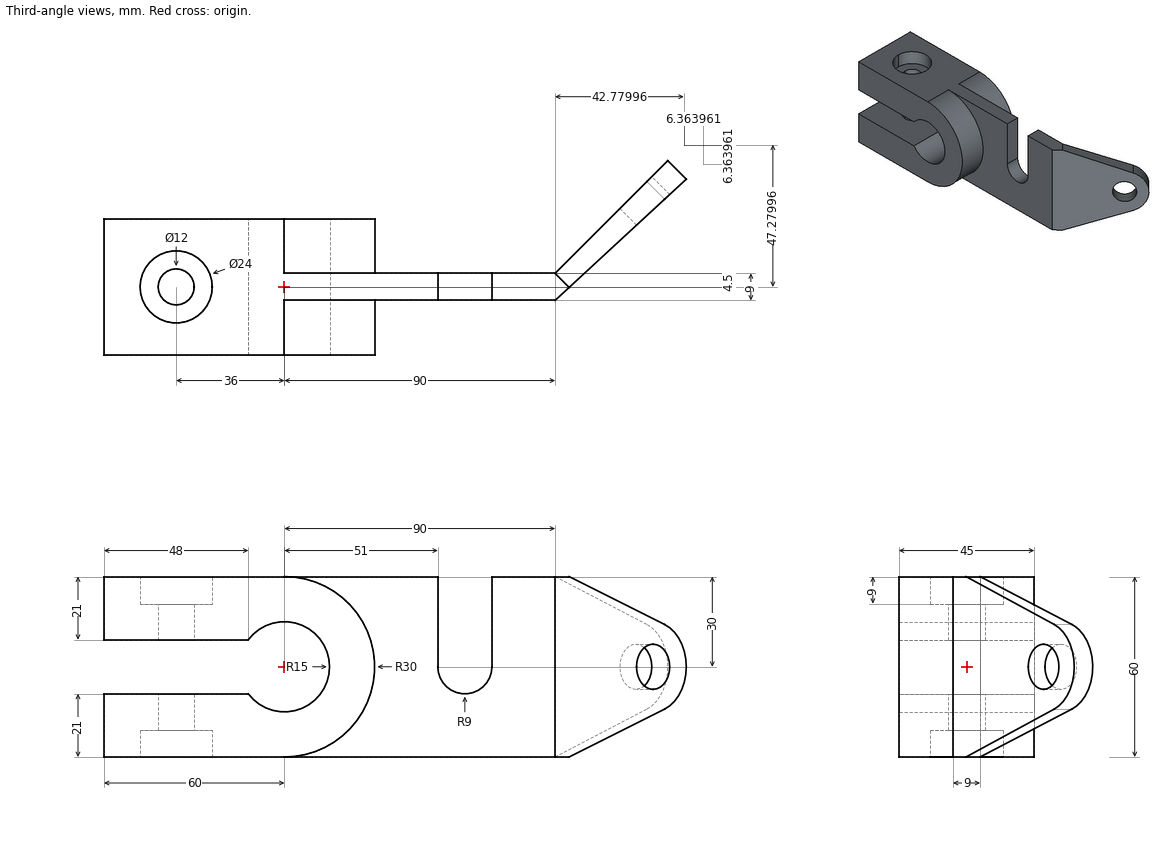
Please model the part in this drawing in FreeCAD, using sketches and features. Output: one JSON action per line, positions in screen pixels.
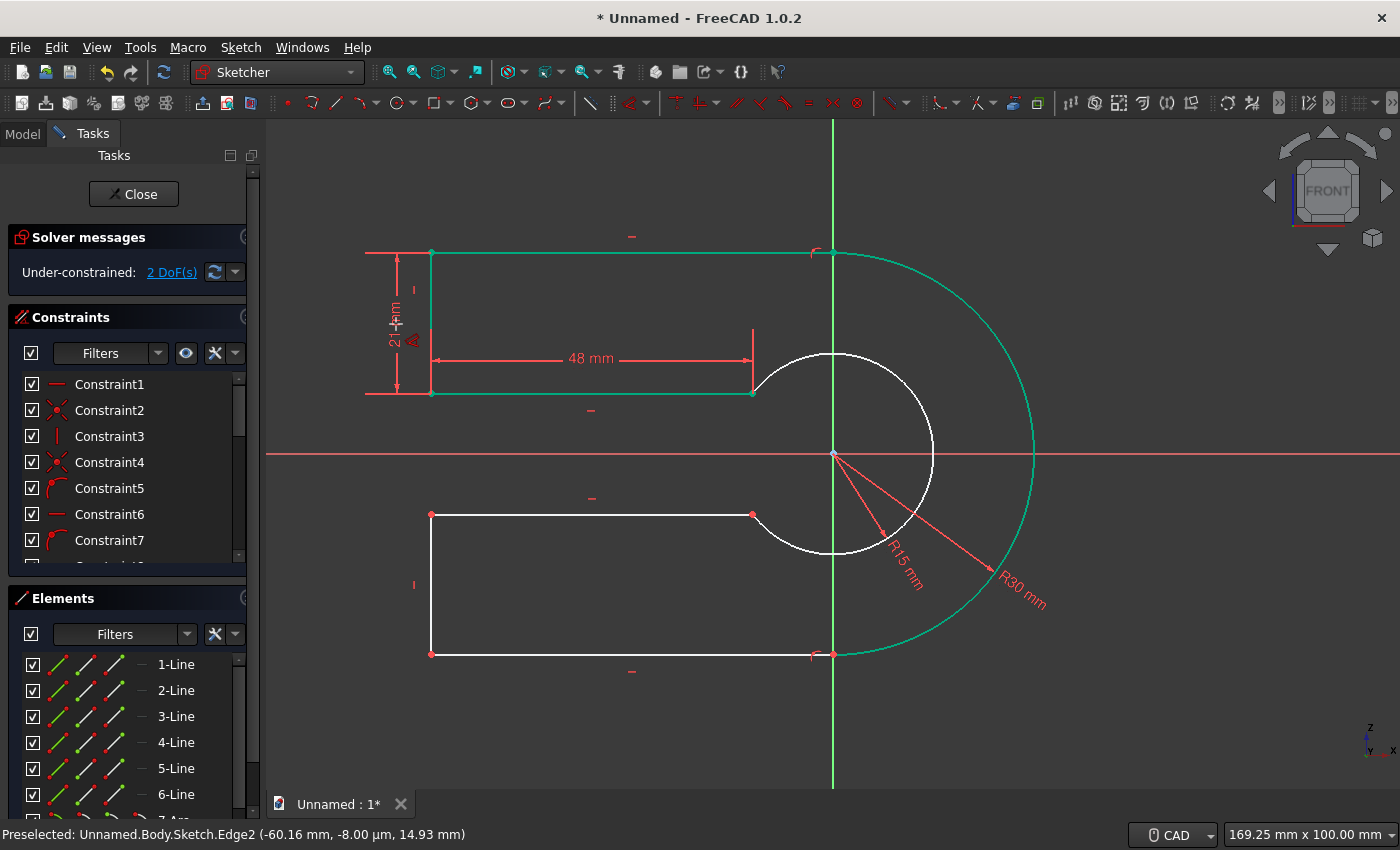
{"action": "left_click", "coordinate": [712, 655]}
{"action": "left_click", "coordinate": [632, 689]}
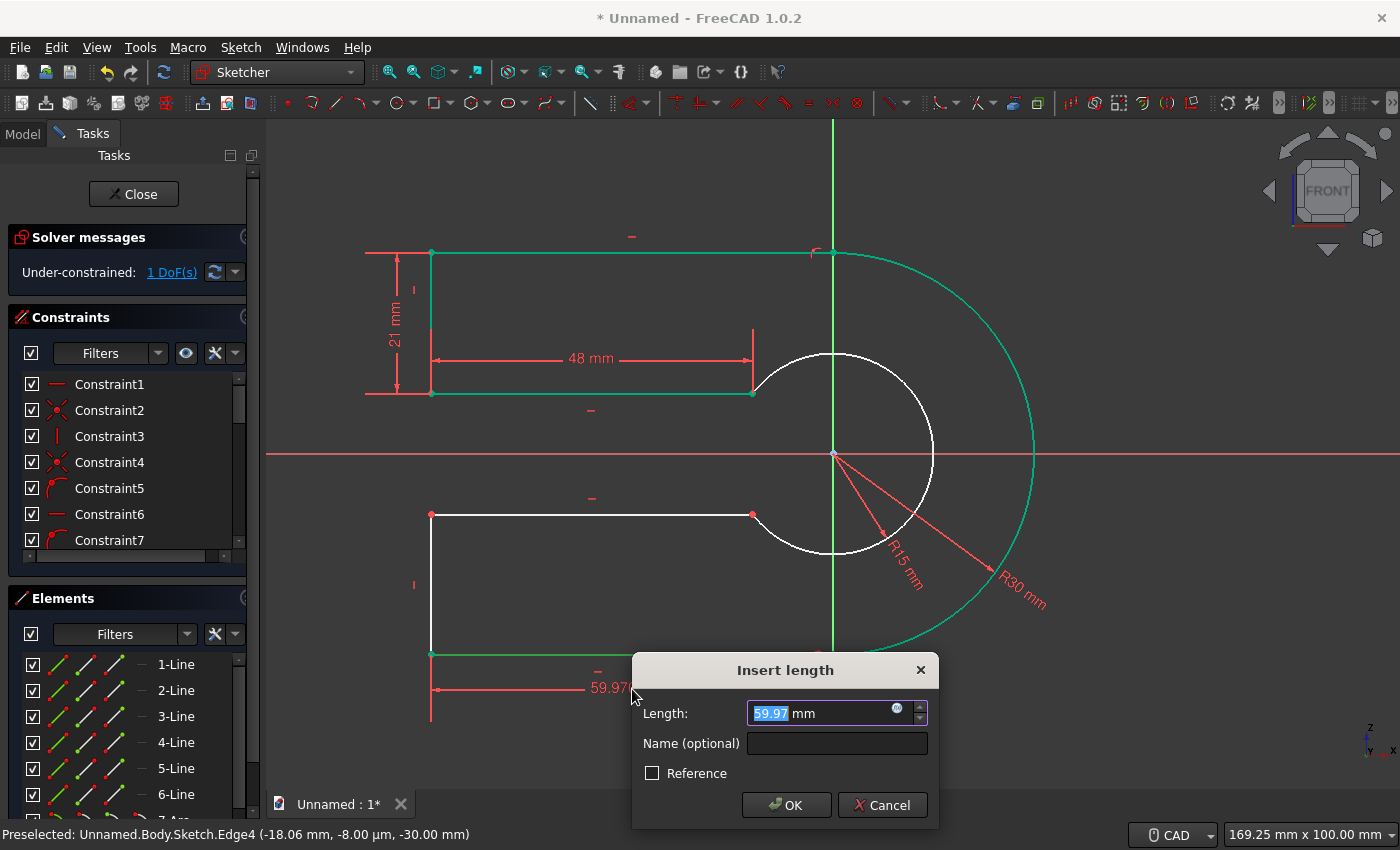
{"action": "type", "text": "60"}
{"action": "key", "text": "Return"}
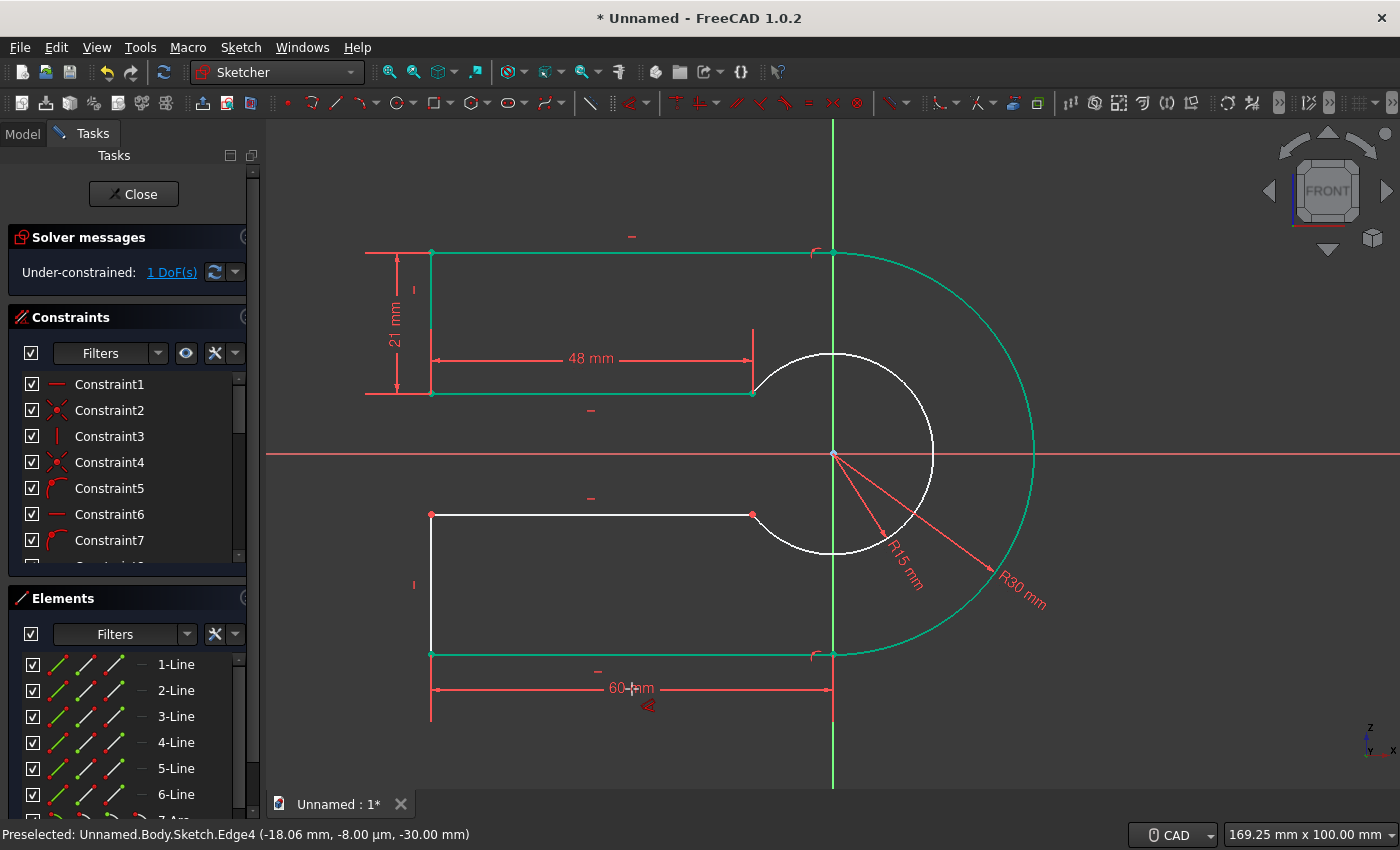
{"action": "left_click", "coordinate": [431, 613]}
{"action": "left_click", "coordinate": [397, 585]}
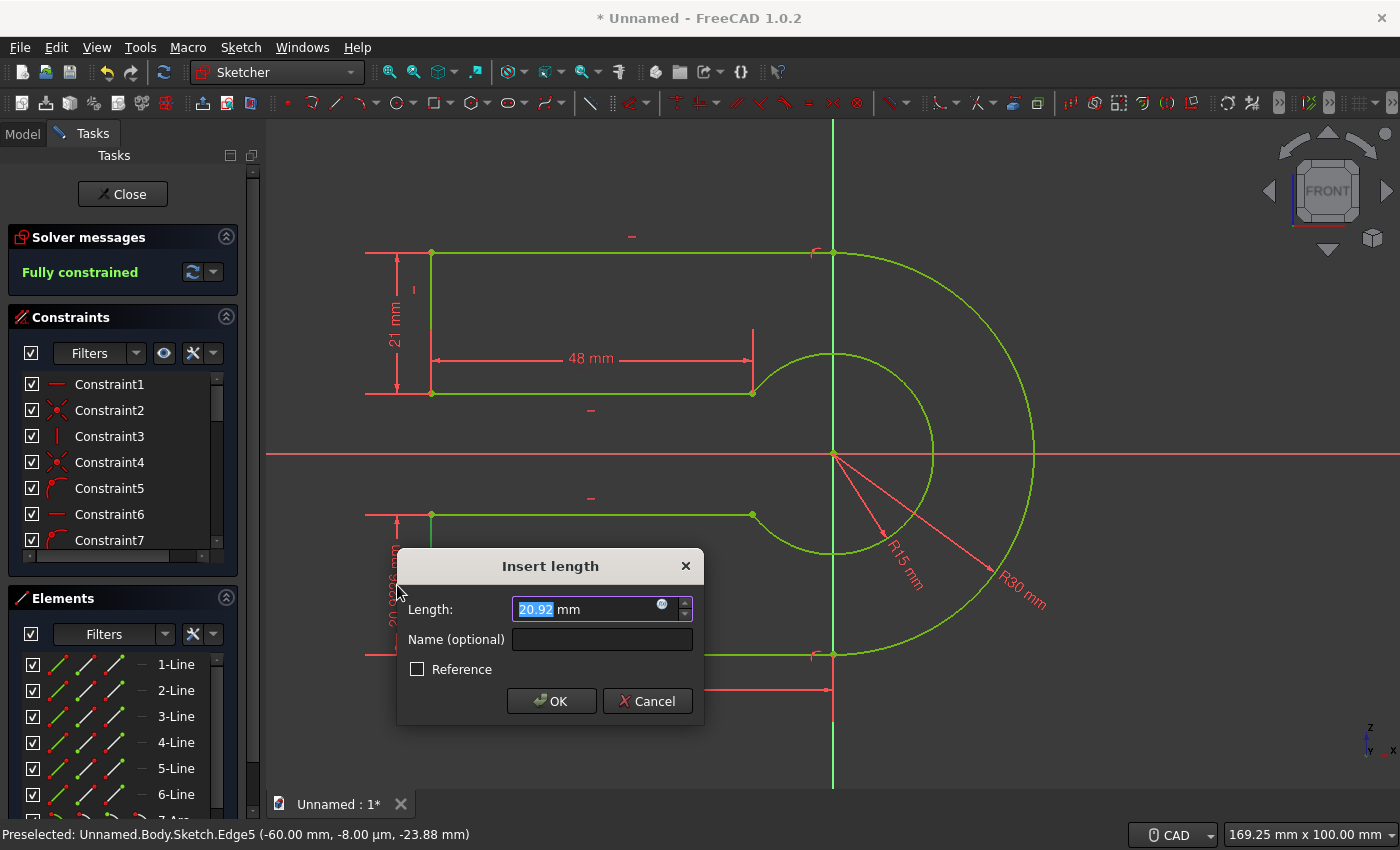
{"action": "type", "text": "21"}
{"action": "key", "text": "Return"}
{"action": "key", "text": "Escape"}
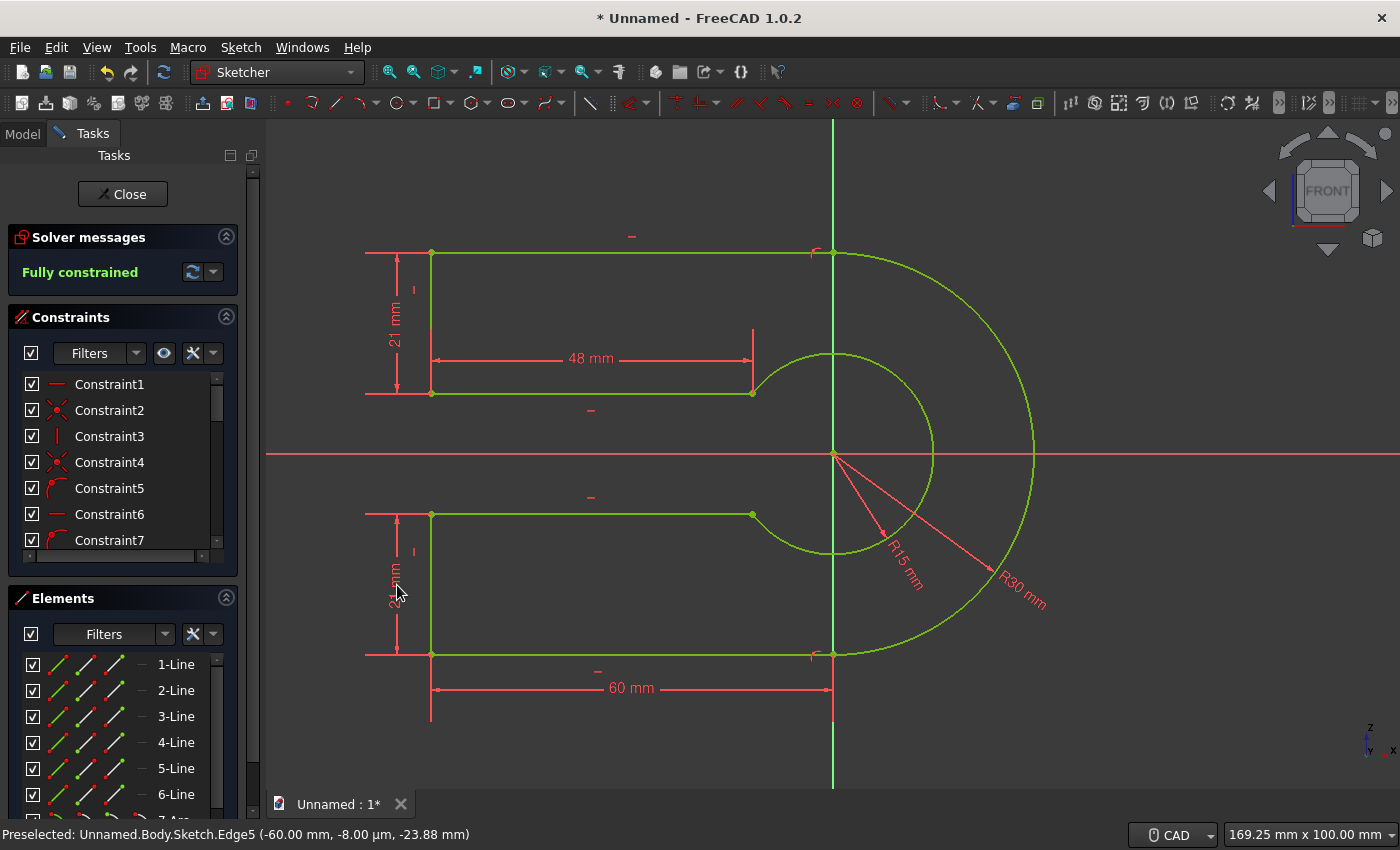
{"action": "left_click", "coordinate": [123, 194]}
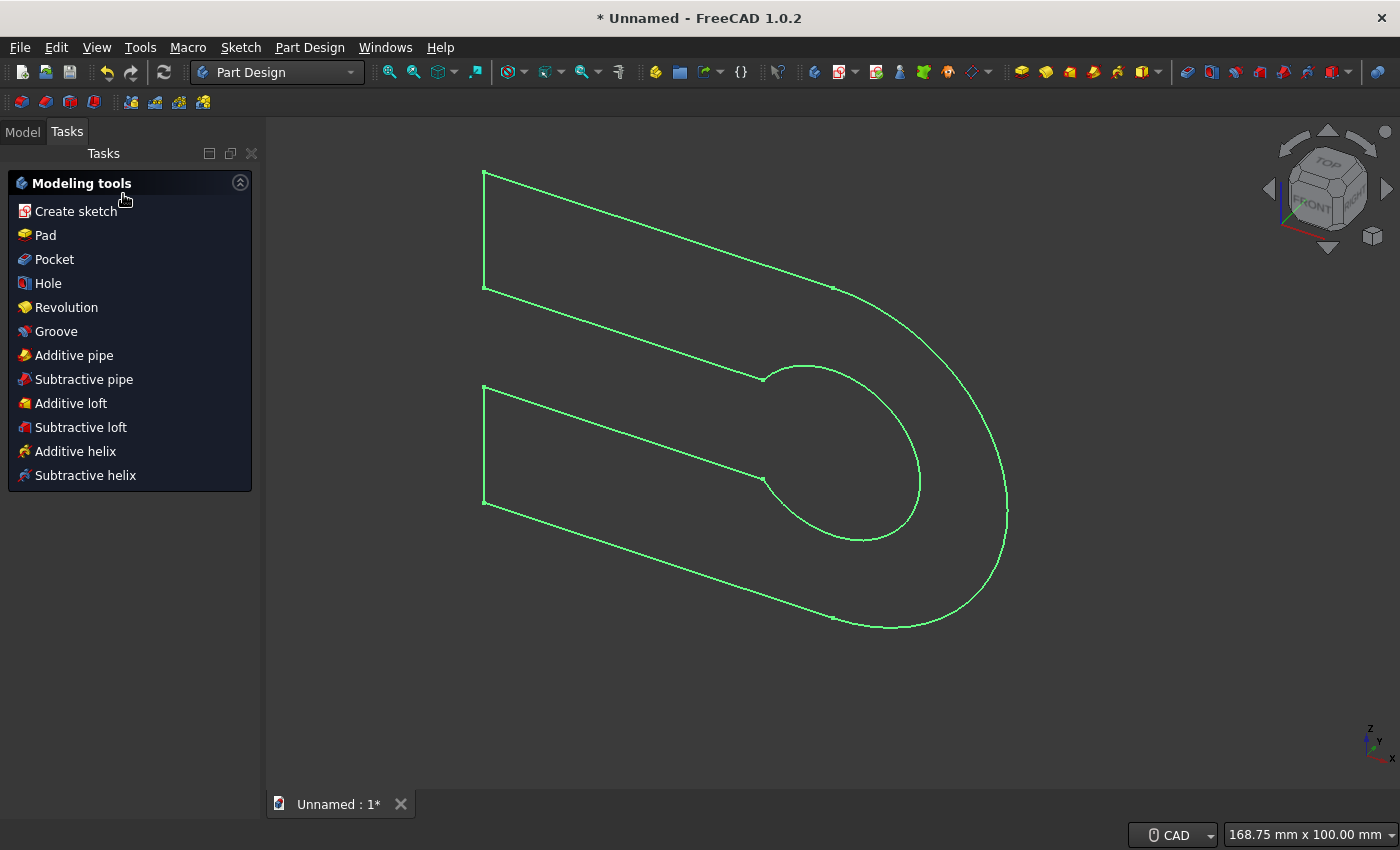
{"action": "left_click", "coordinate": [1022, 72]}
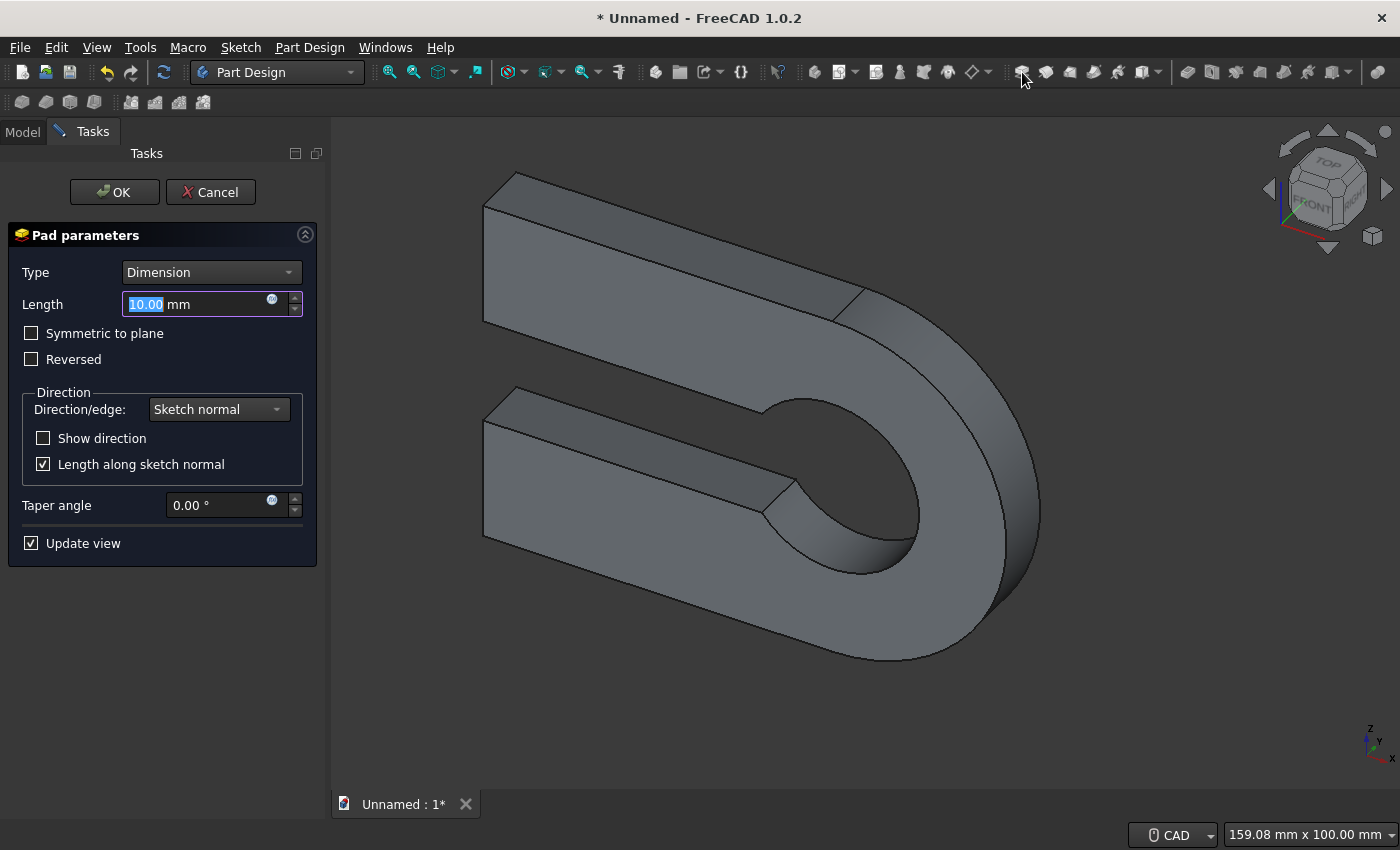
{"action": "type", "text": "45"}
{"action": "key", "text": "Tab"}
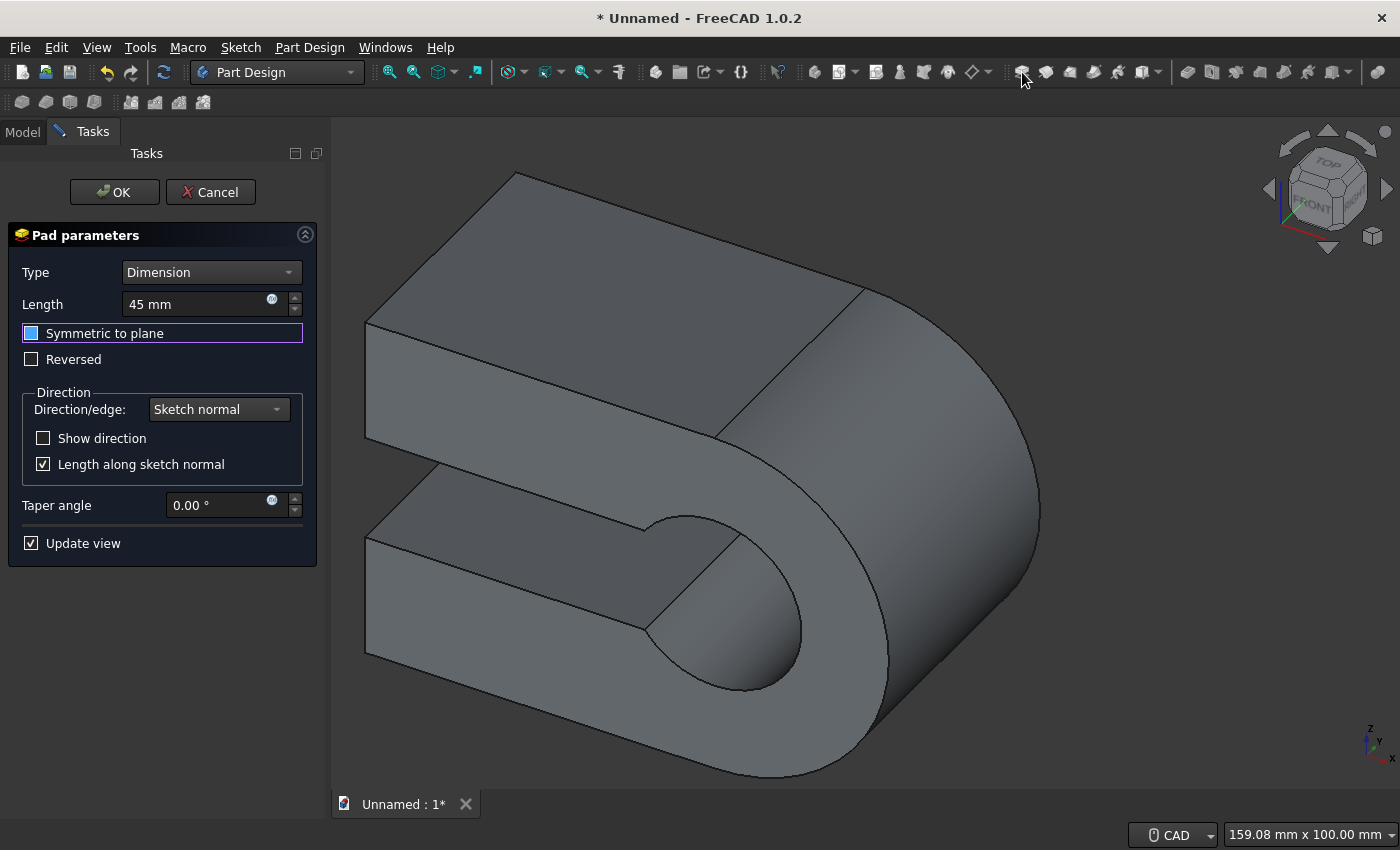
{"action": "left_click", "coordinate": [30, 333]}